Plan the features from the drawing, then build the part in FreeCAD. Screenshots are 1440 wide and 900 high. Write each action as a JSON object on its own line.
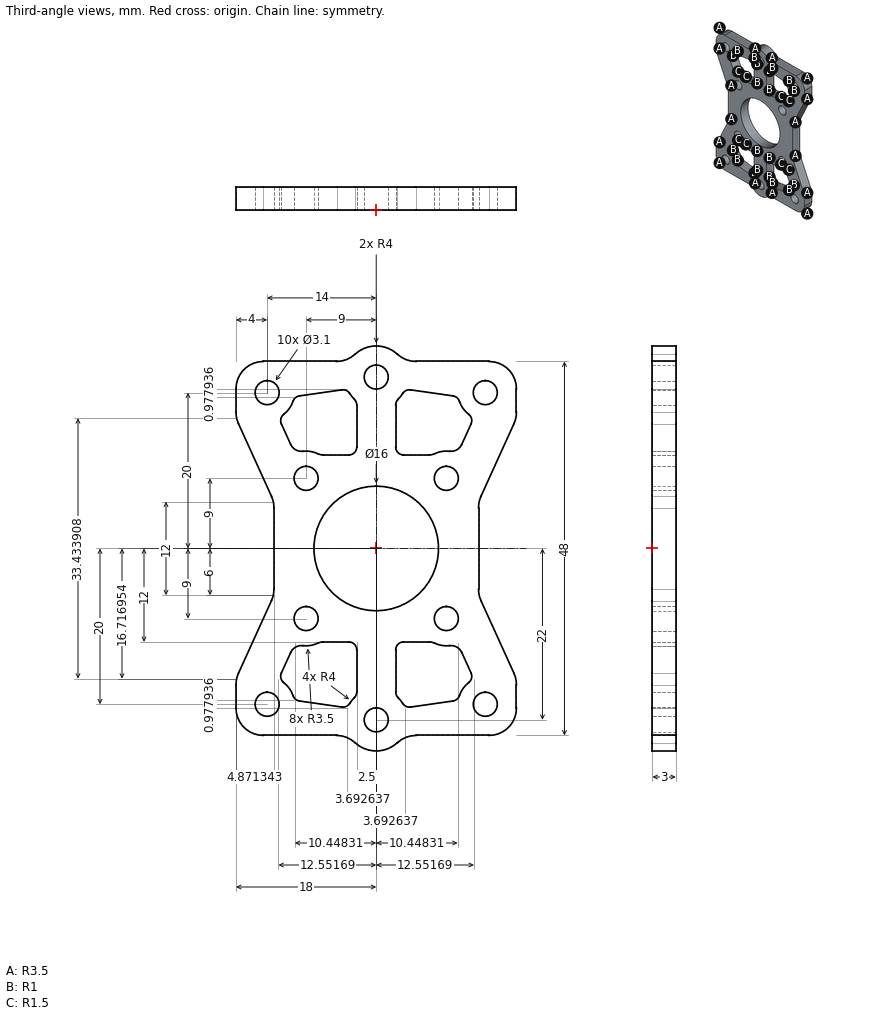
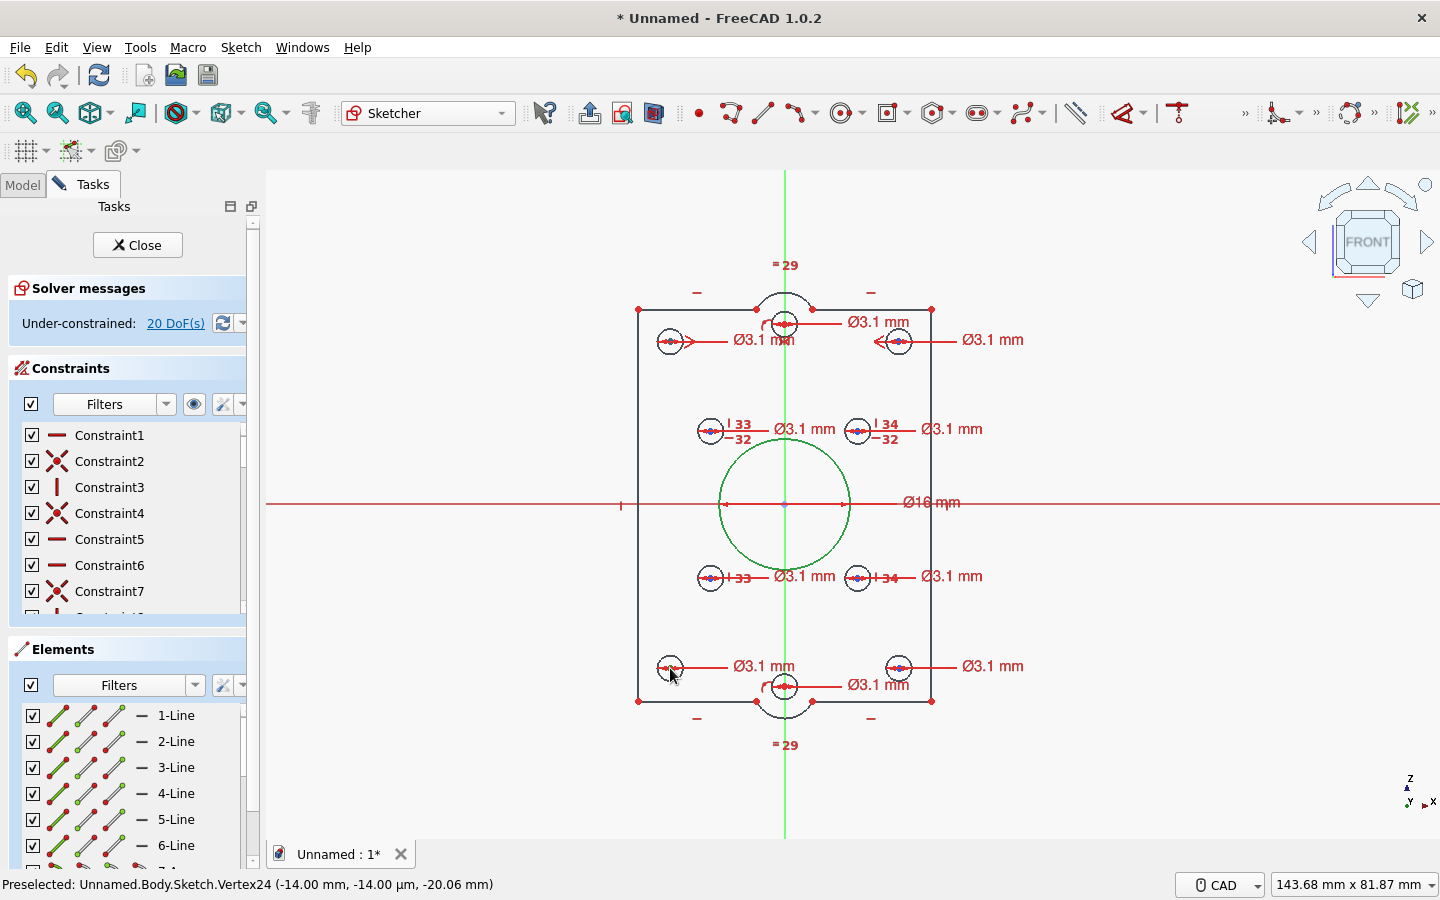
{"action": "left_click", "coordinate": [364, 504]}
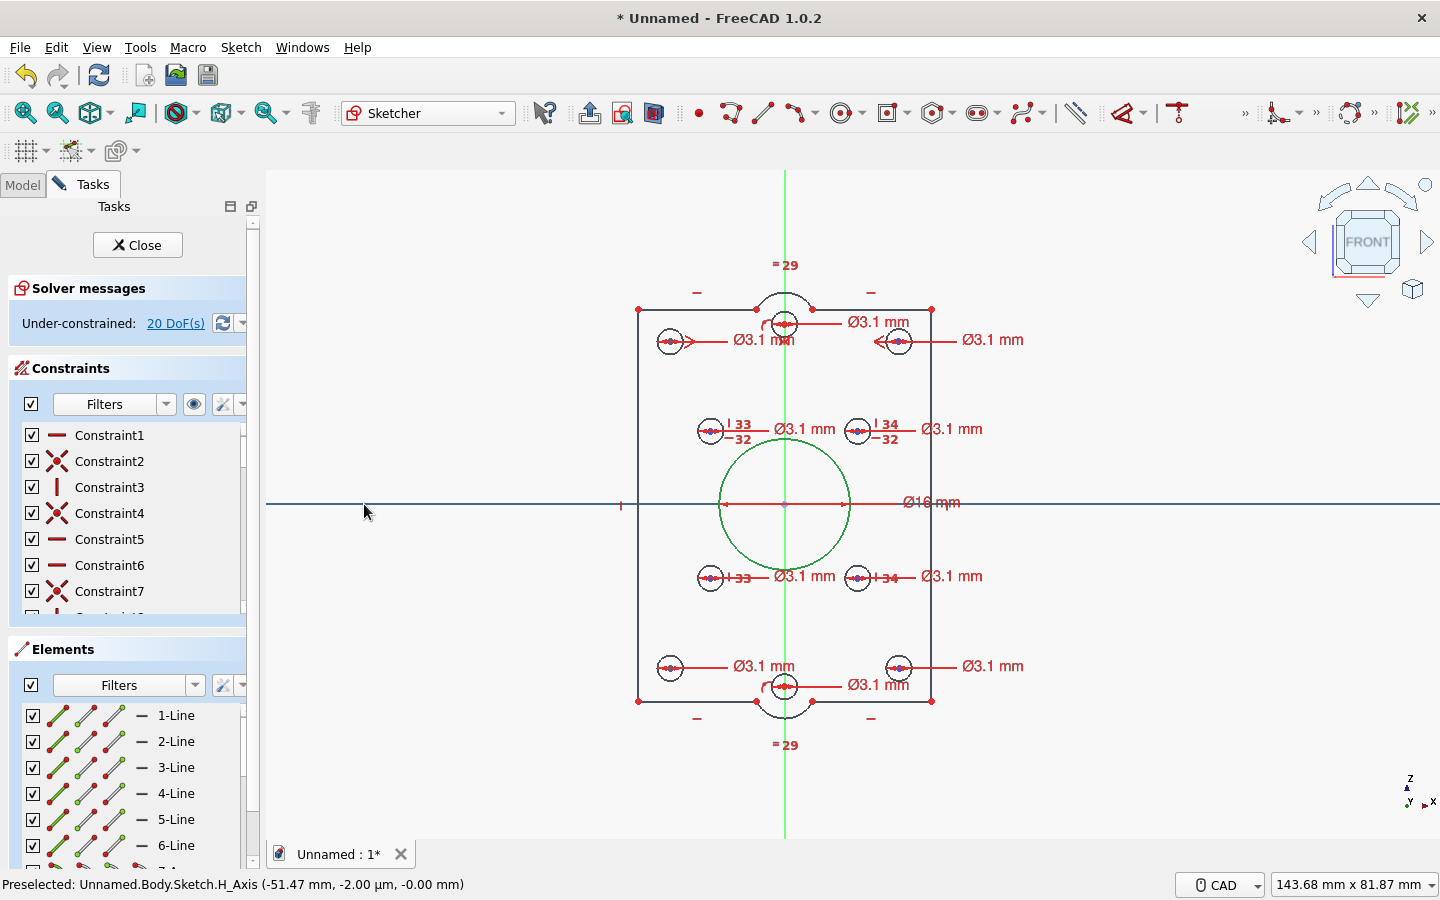
{"action": "key", "text": "s"}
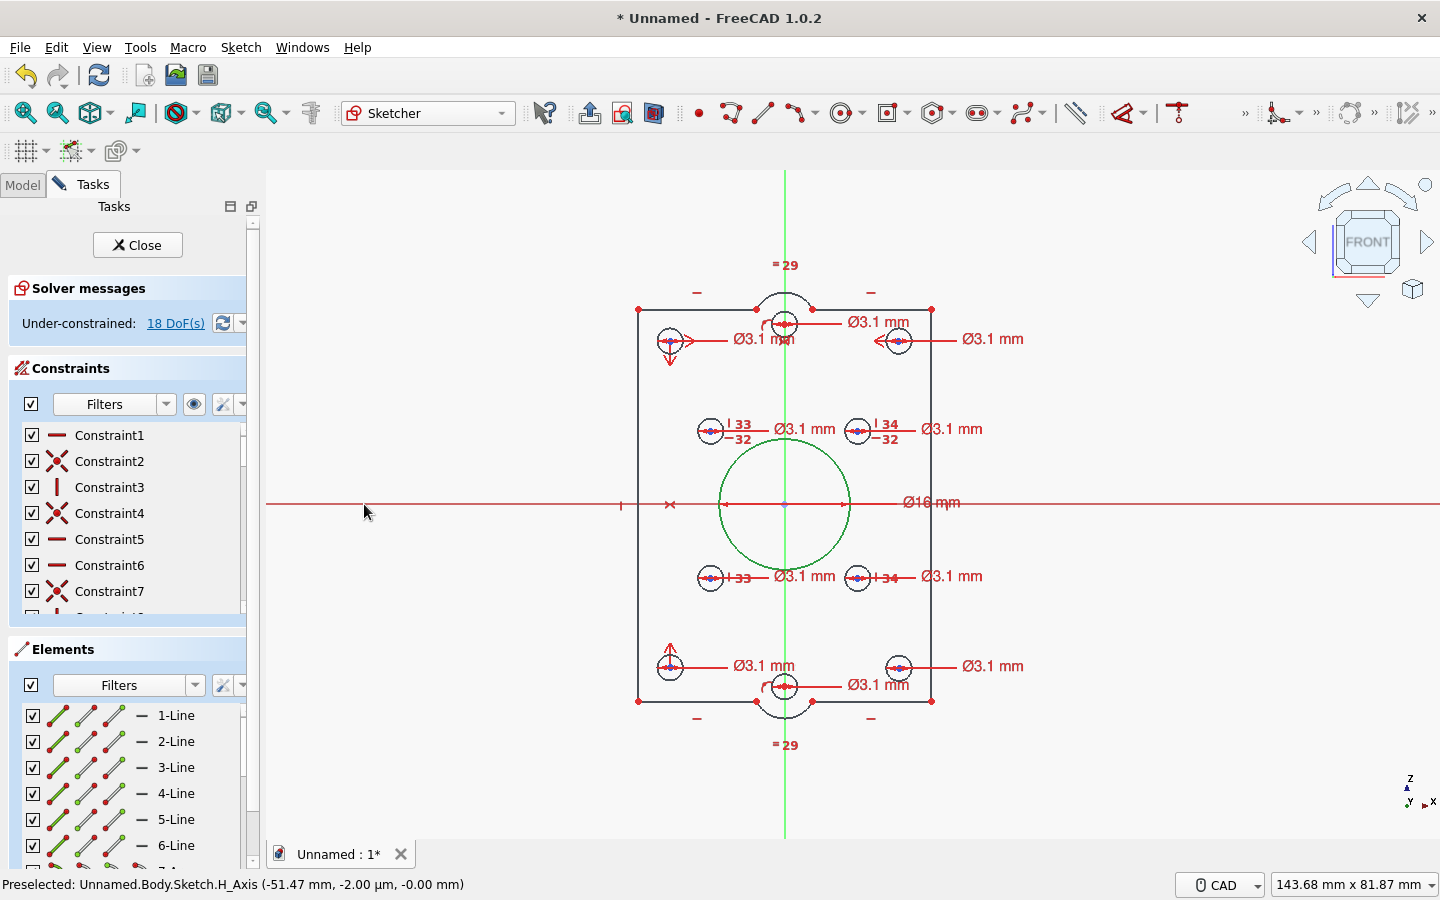
{"action": "left_click", "coordinate": [711, 578]}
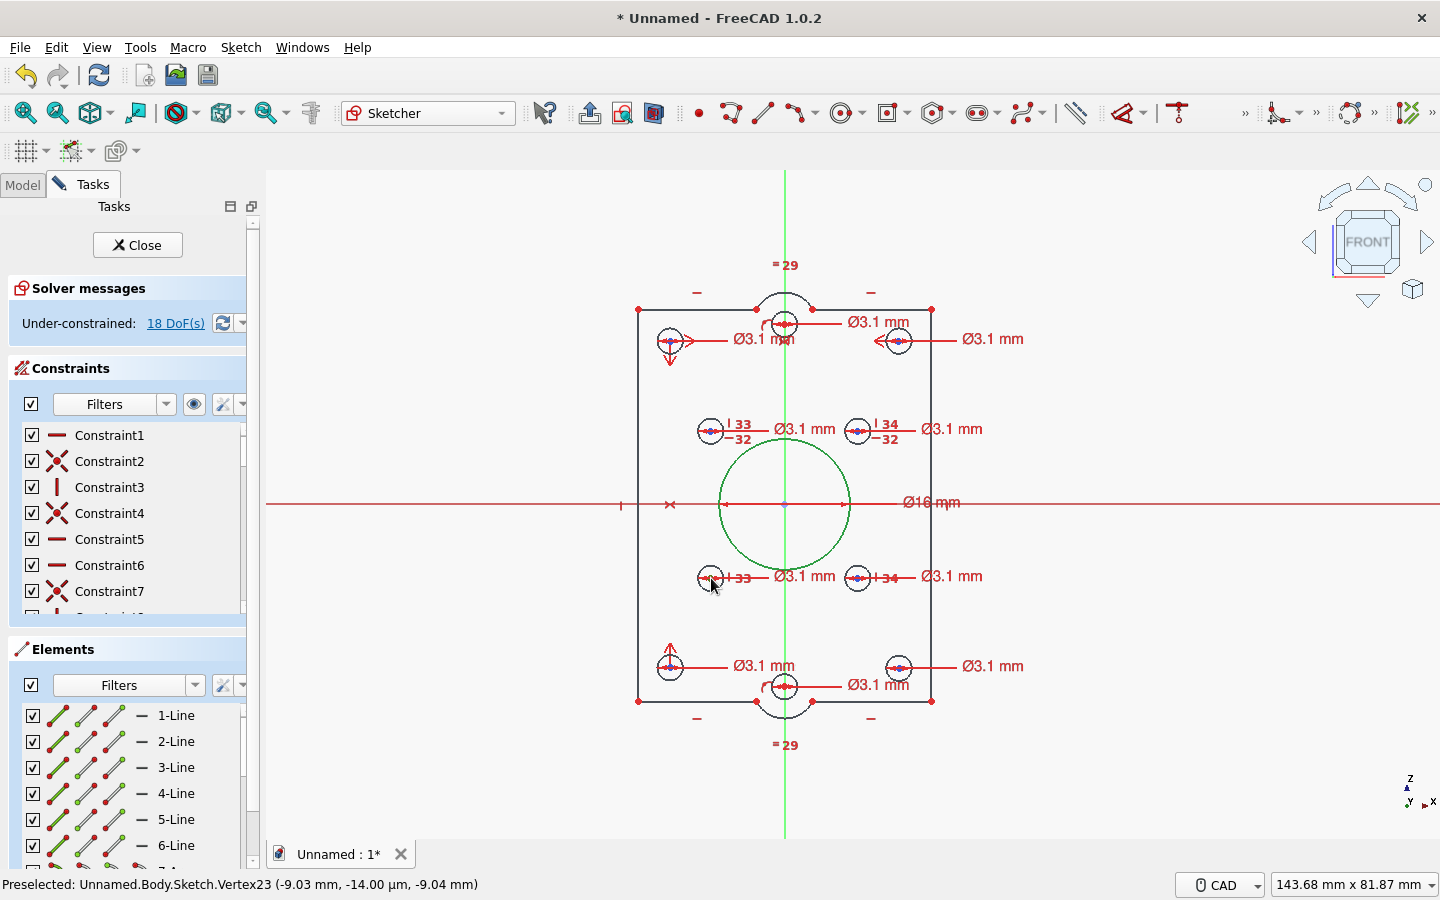
{"action": "left_click", "coordinate": [858, 578]}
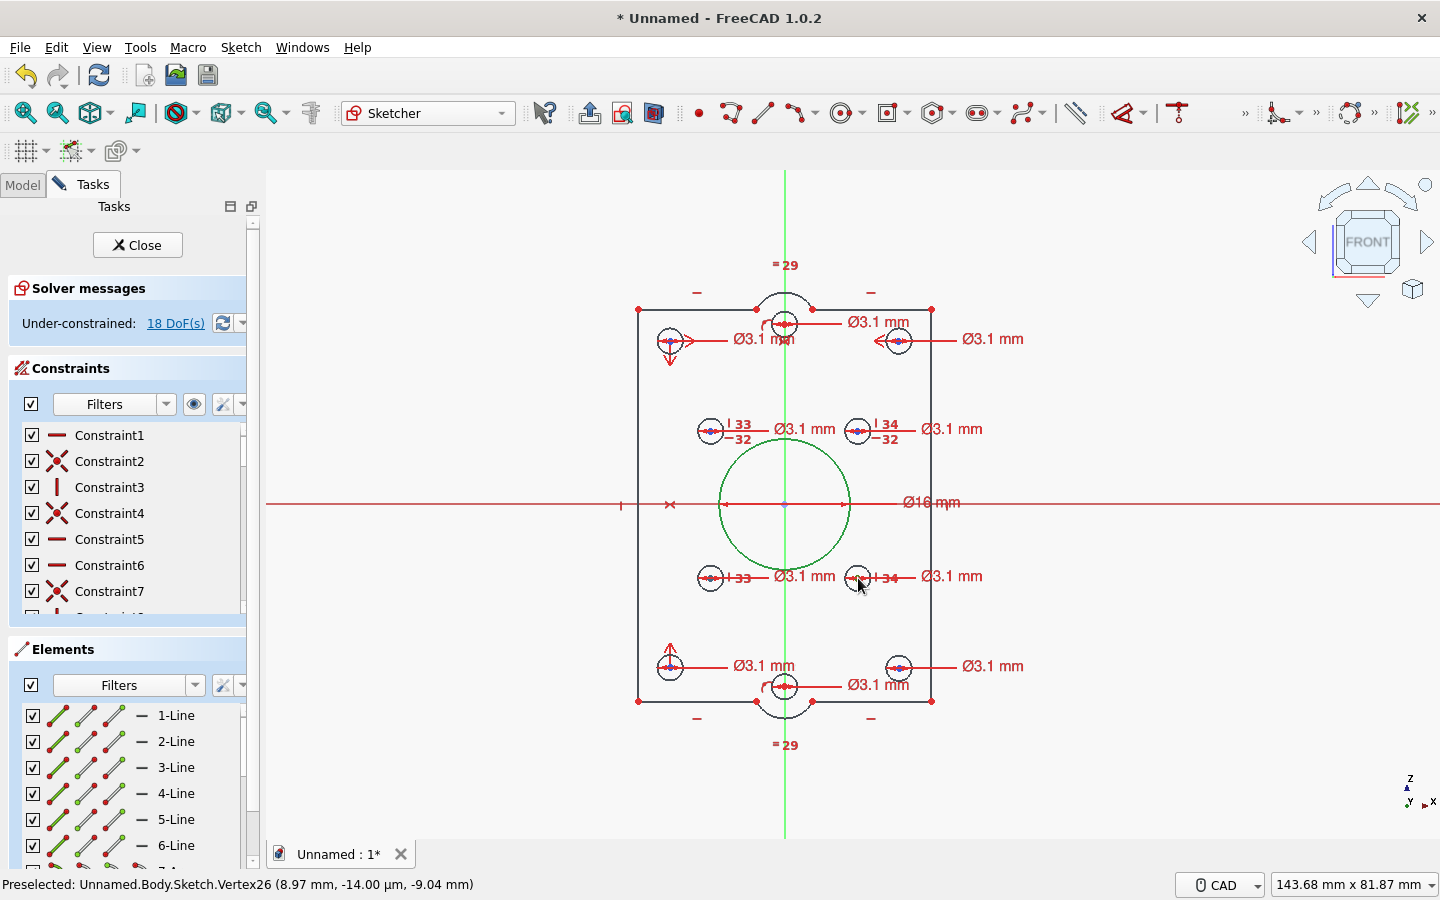
{"action": "left_click", "coordinate": [785, 767]}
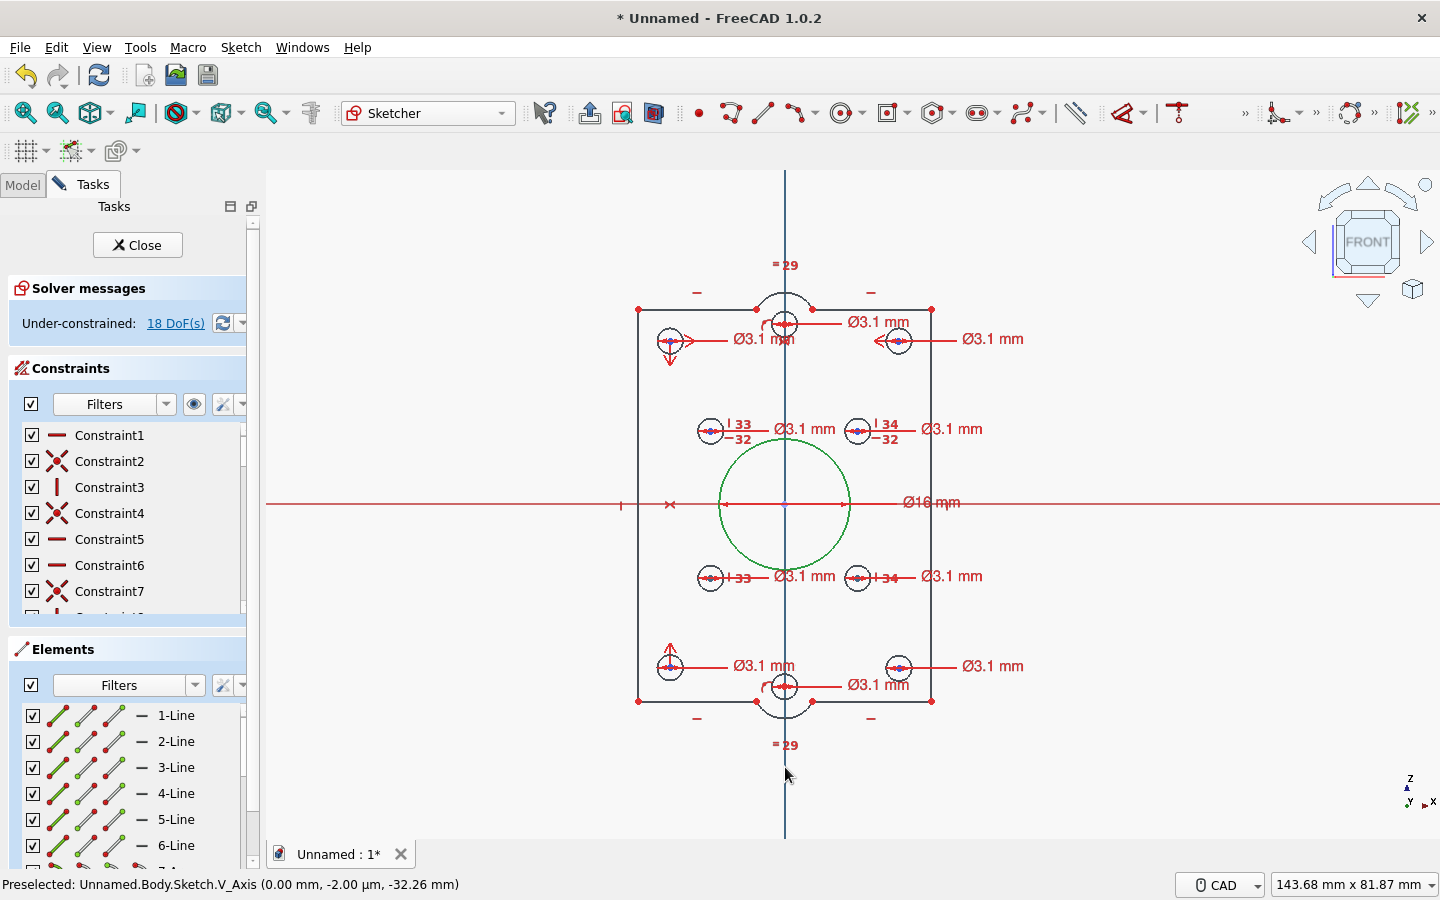
{"action": "key", "text": "s"}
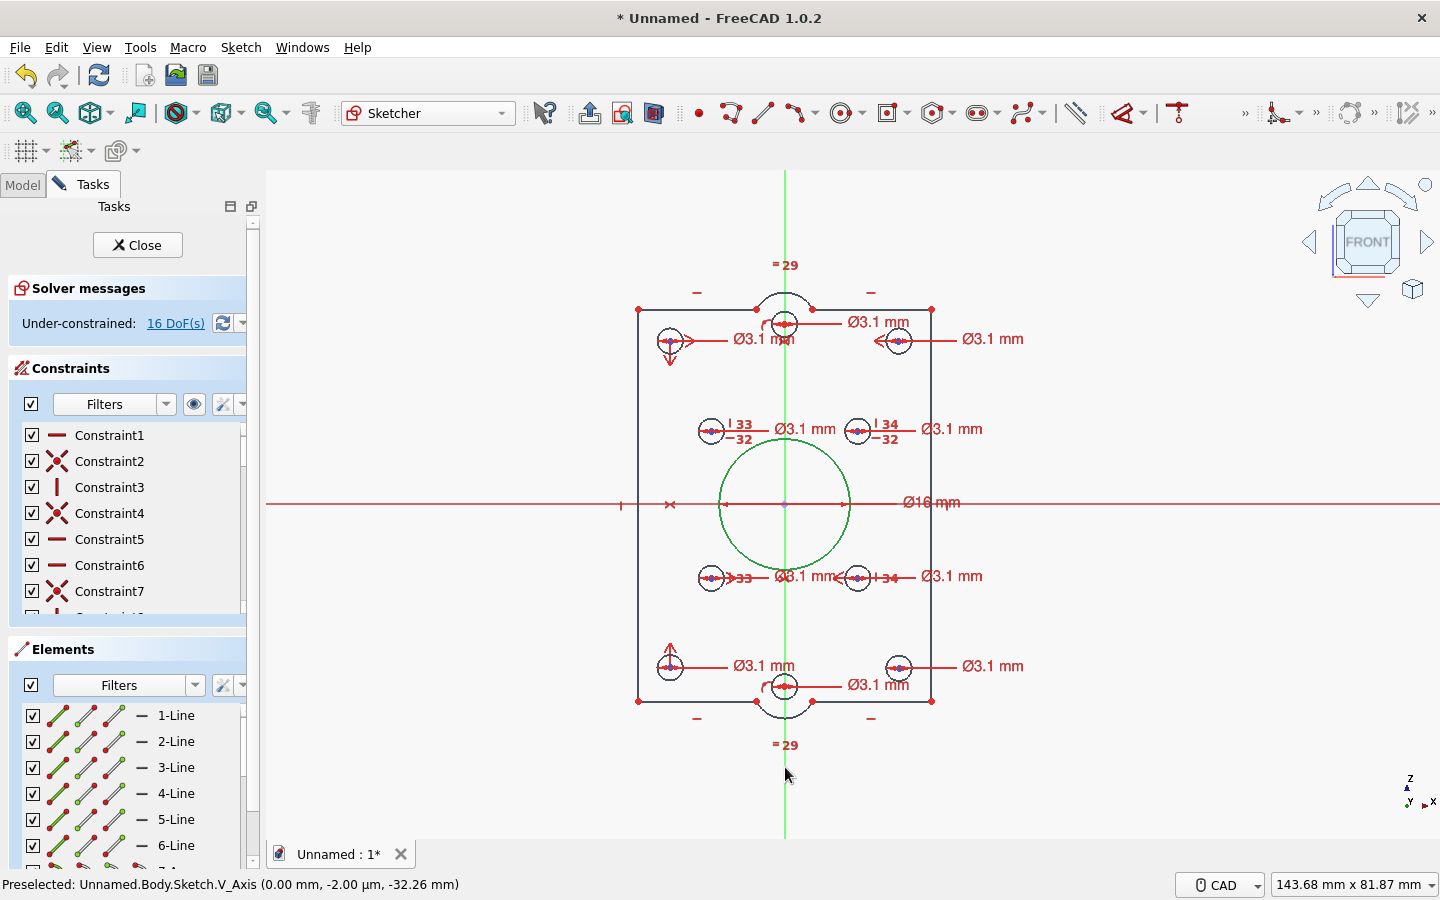
{"action": "left_click", "coordinate": [899, 341]}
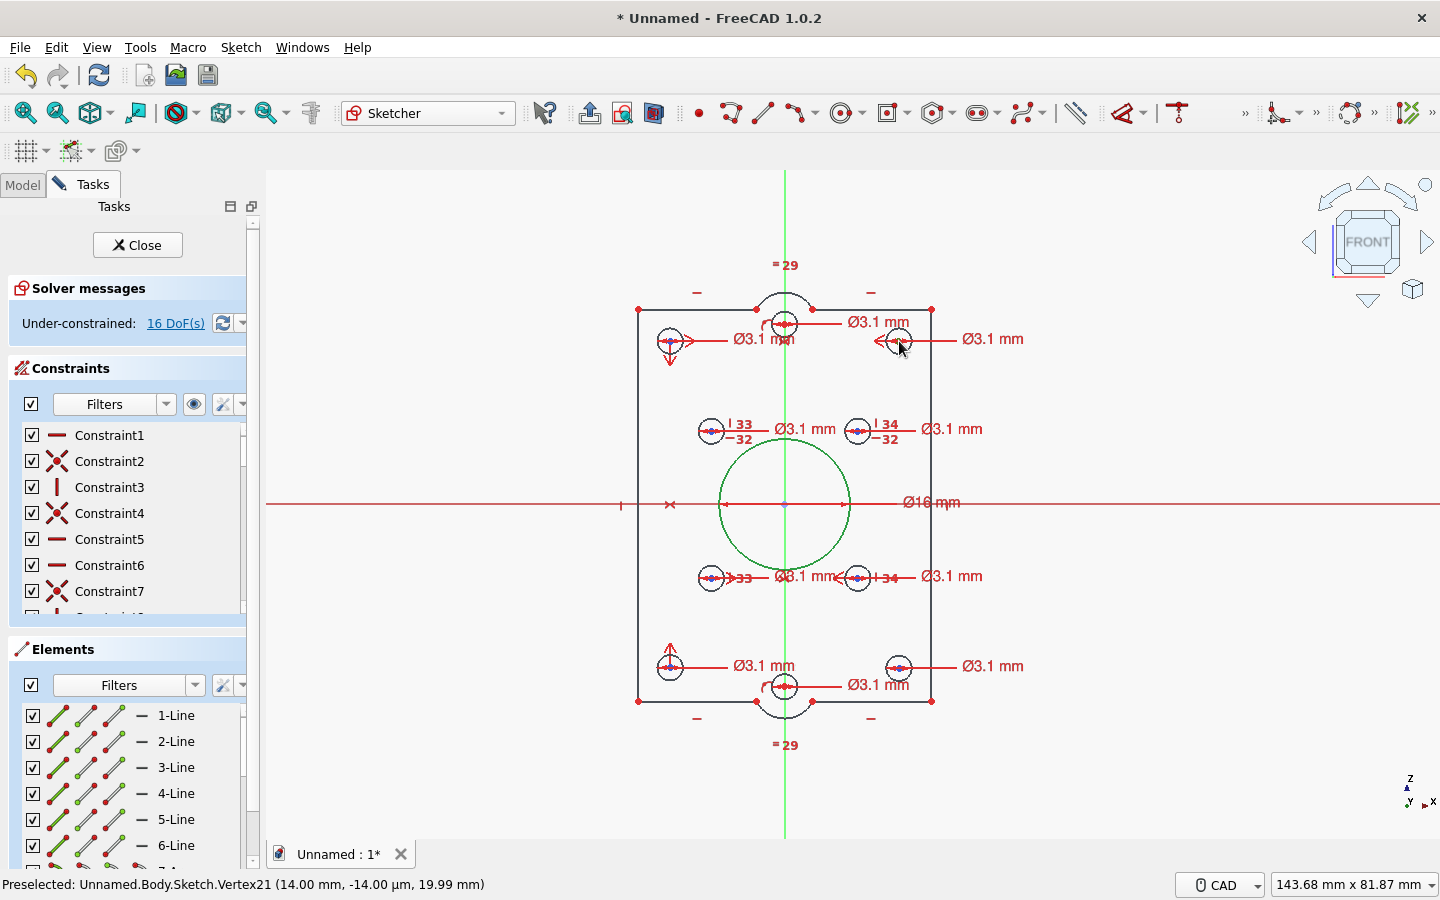
{"action": "left_click", "coordinate": [899, 668]}